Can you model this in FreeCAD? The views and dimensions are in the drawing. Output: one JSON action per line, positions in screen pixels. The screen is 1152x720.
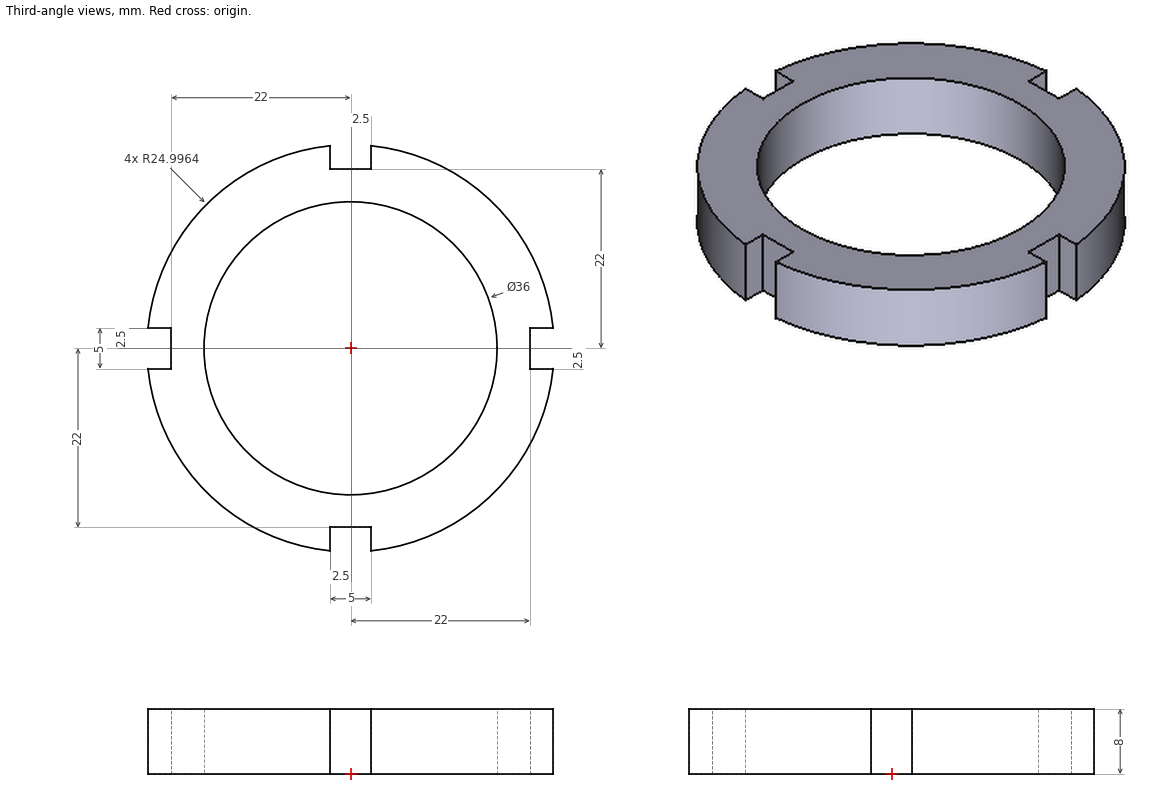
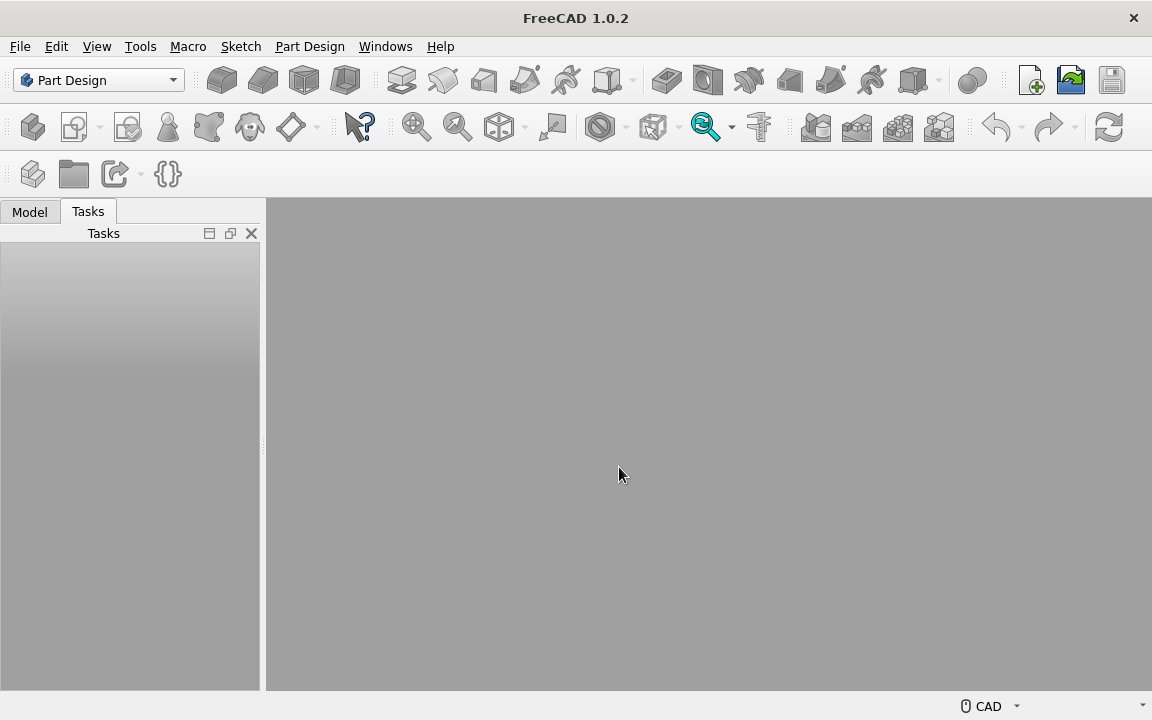
{"action": "key", "text": "ctrl+n"}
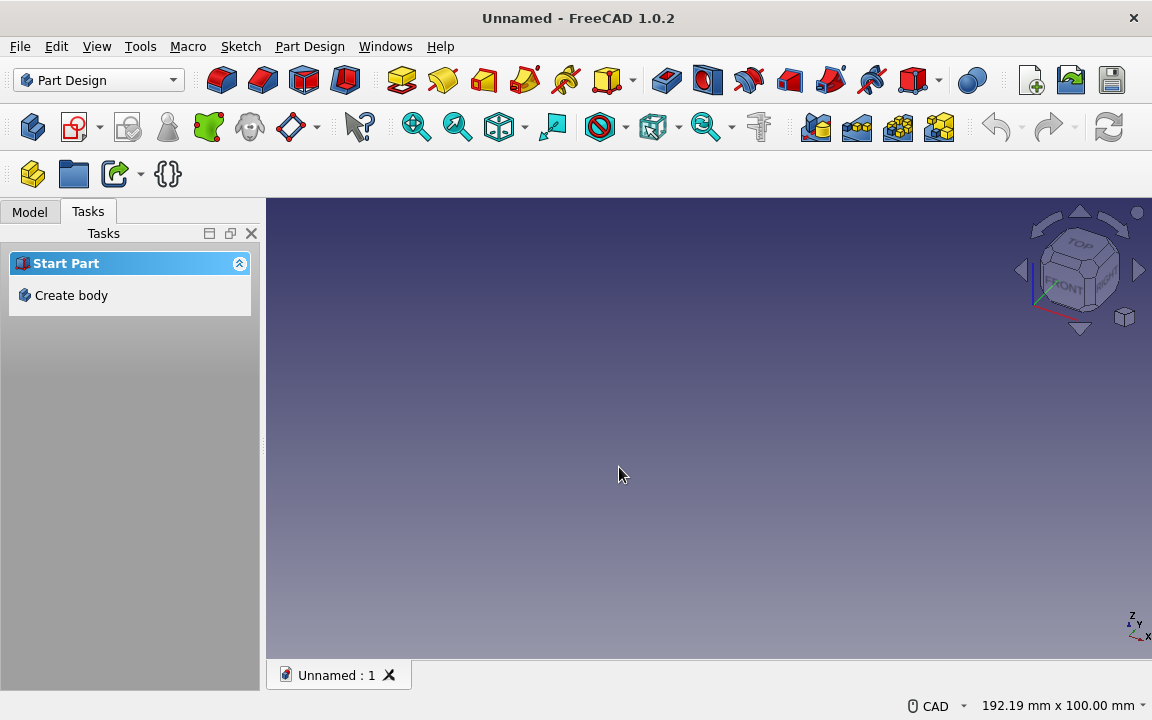
{"action": "left_click", "coordinate": [74, 128]}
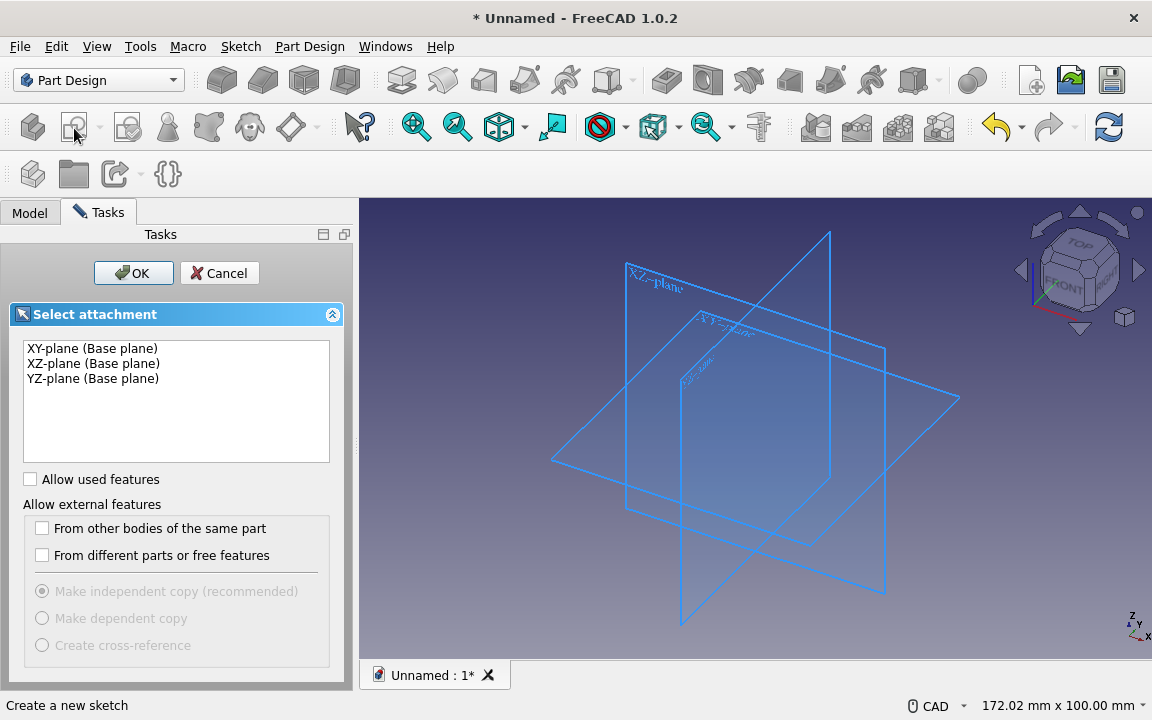
{"action": "left_click", "coordinate": [84, 348]}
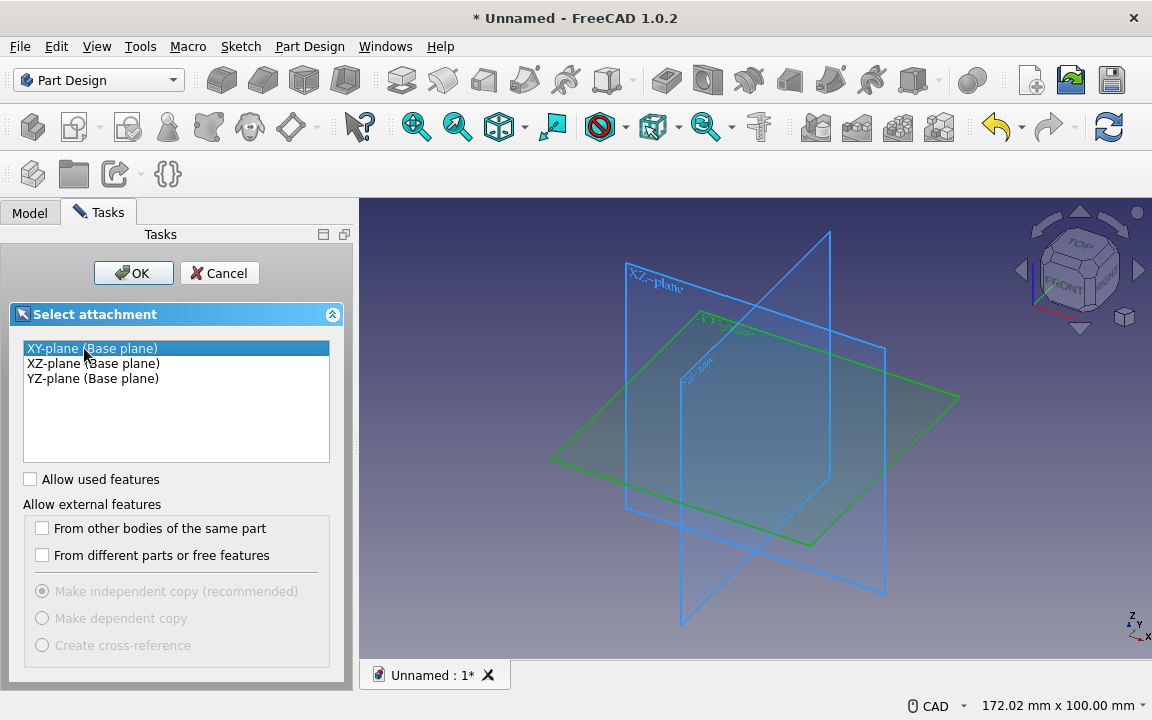
{"action": "left_click", "coordinate": [134, 273]}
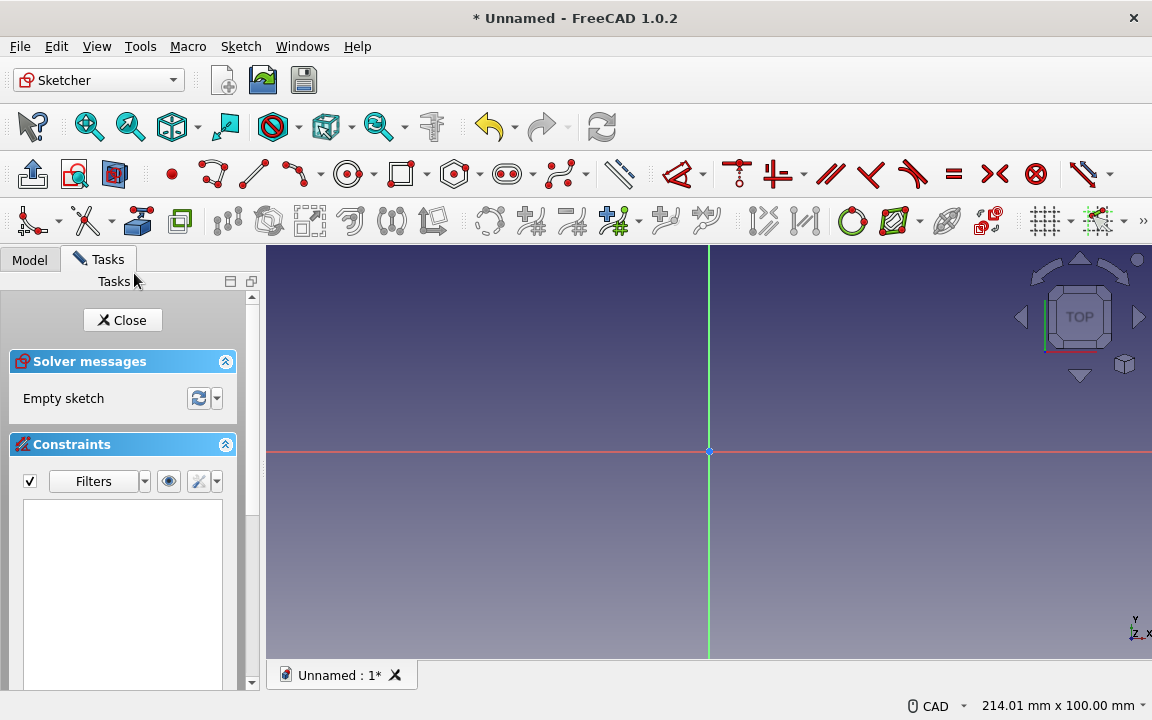
{"action": "key", "text": "g m"}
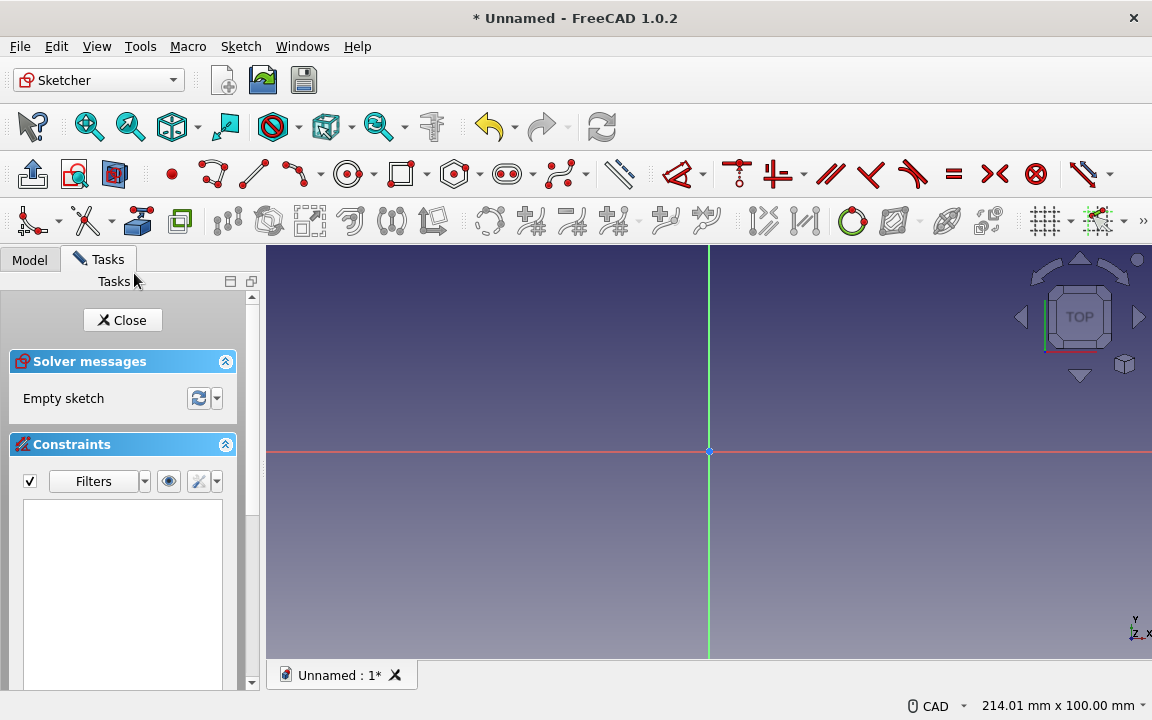
{"action": "scroll", "coordinate": [606, 442], "scroll_direction": "up", "scroll_amount": 3}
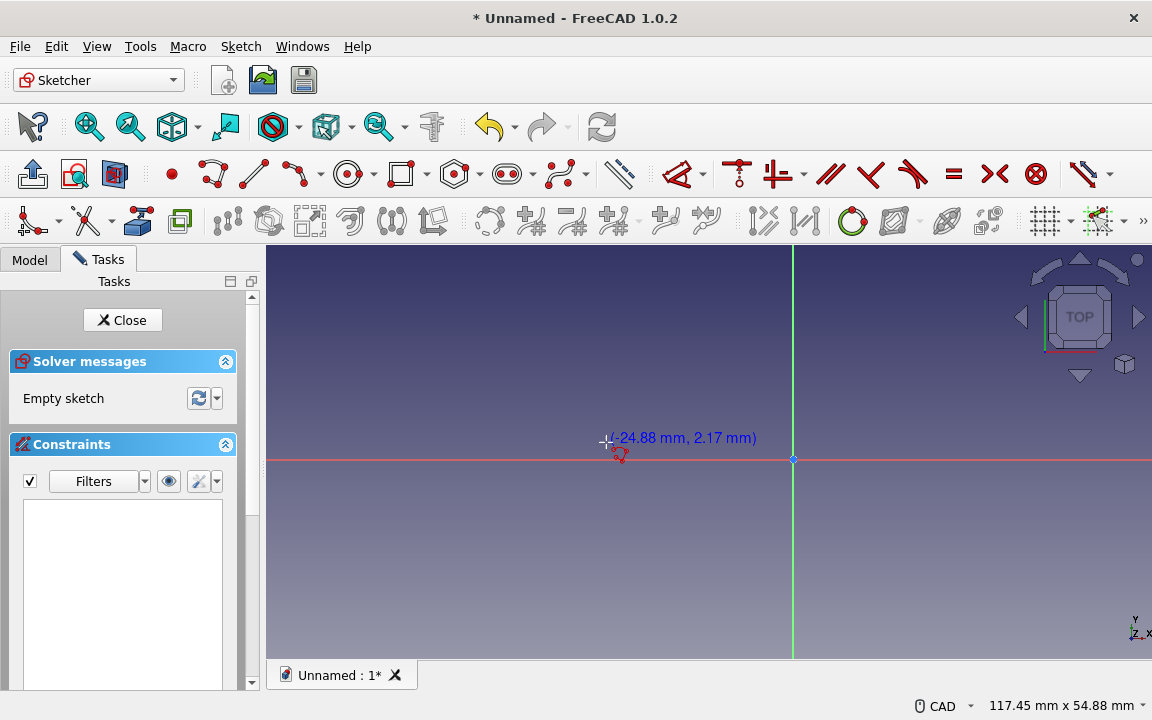
{"action": "left_click", "coordinate": [606, 441]}
{"action": "left_click", "coordinate": [627, 441]}
{"action": "left_click", "coordinate": [627, 479]}
{"action": "left_click", "coordinate": [606, 479]}
{"action": "right_click", "coordinate": [606, 479]}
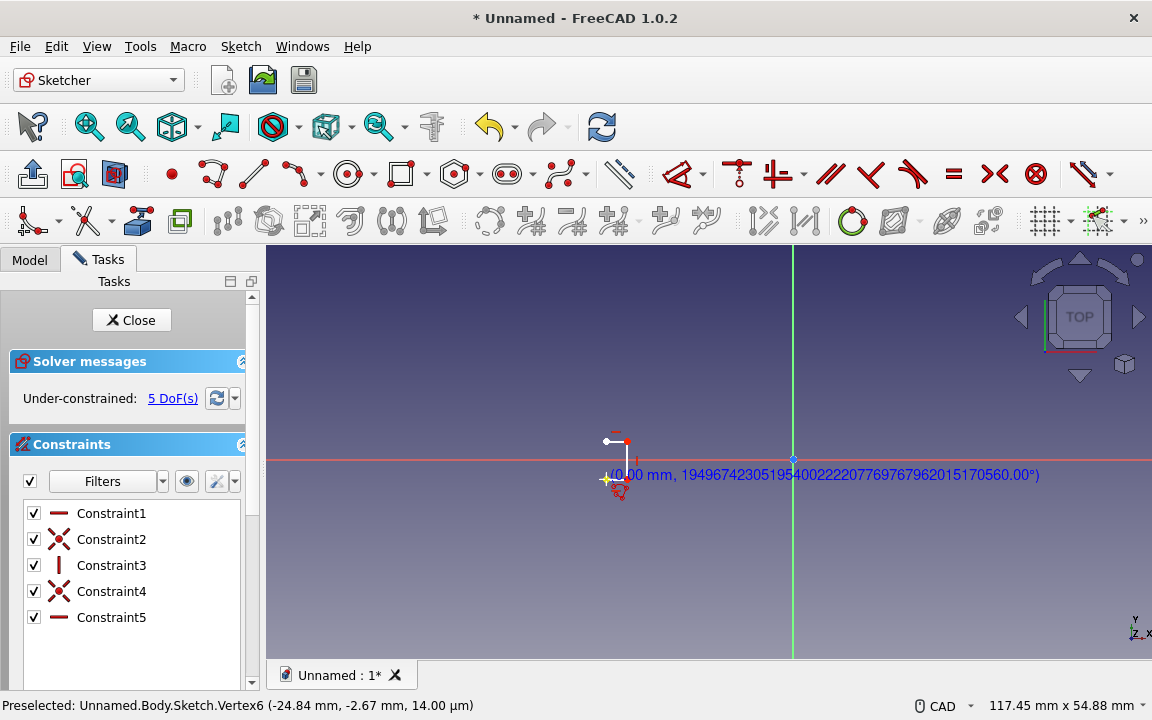
{"action": "scroll", "coordinate": [330, 436], "scroll_direction": "down", "scroll_amount": 2}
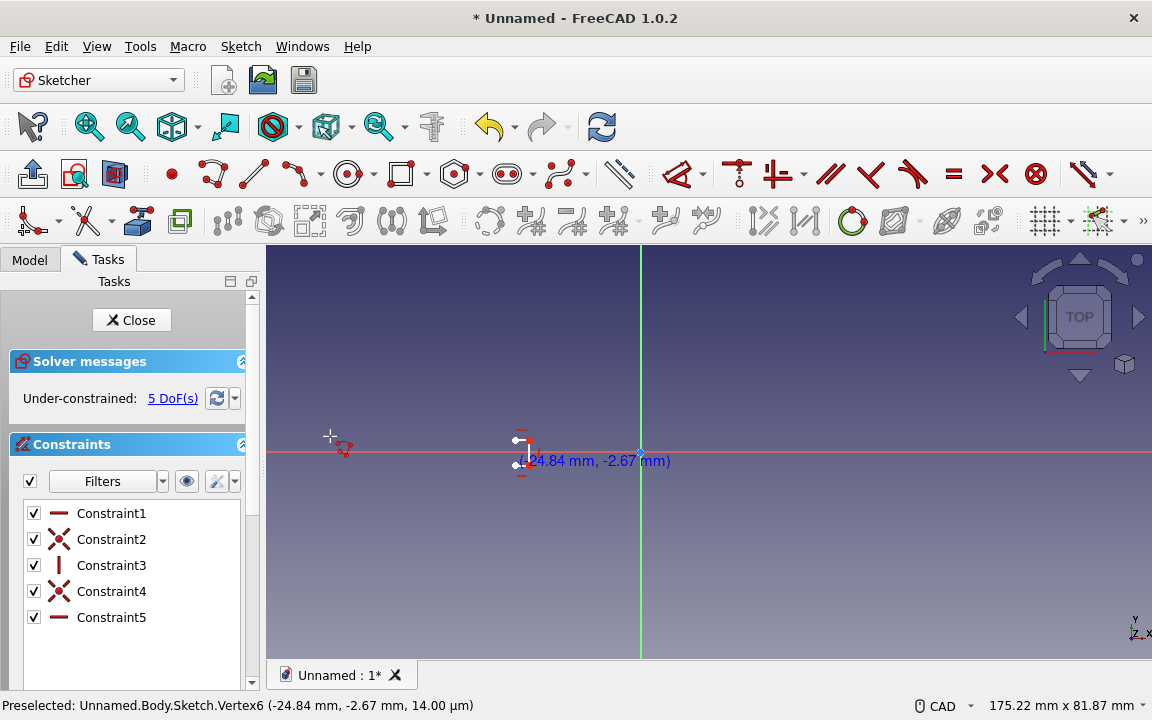
{"action": "scroll", "coordinate": [628, 578], "scroll_direction": "up", "scroll_amount": 2}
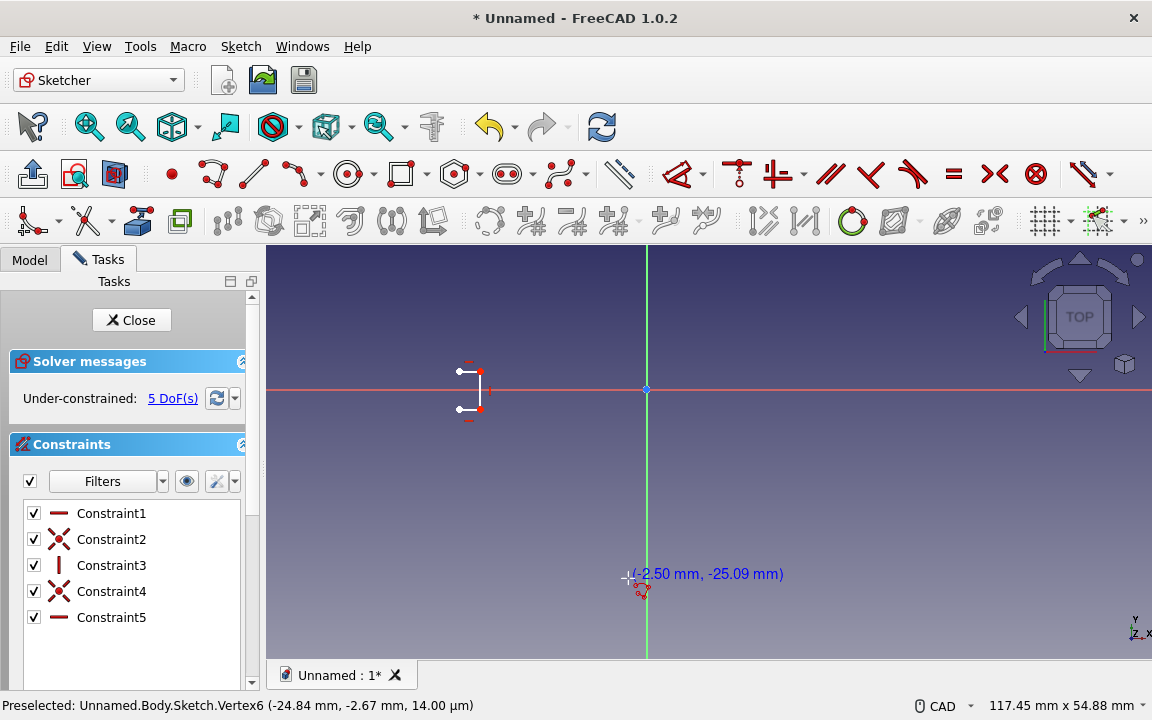
{"action": "left_click", "coordinate": [628, 577]}
{"action": "left_click", "coordinate": [628, 556]}
{"action": "left_click", "coordinate": [665, 556]}
{"action": "left_click", "coordinate": [665, 577]}
{"action": "right_click", "coordinate": [665, 577]}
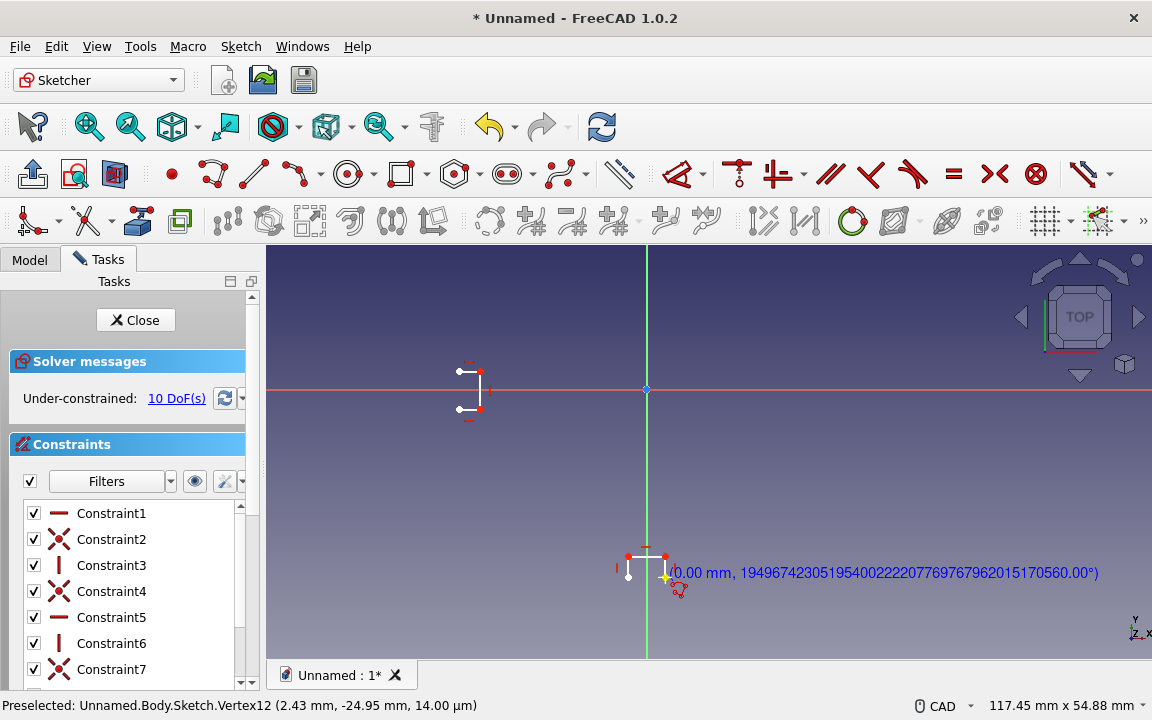
{"action": "left_click", "coordinate": [834, 409]}
{"action": "left_click", "coordinate": [813, 409]}
{"action": "left_click", "coordinate": [813, 371]}
{"action": "left_click", "coordinate": [834, 371]}
{"action": "right_click", "coordinate": [834, 371]}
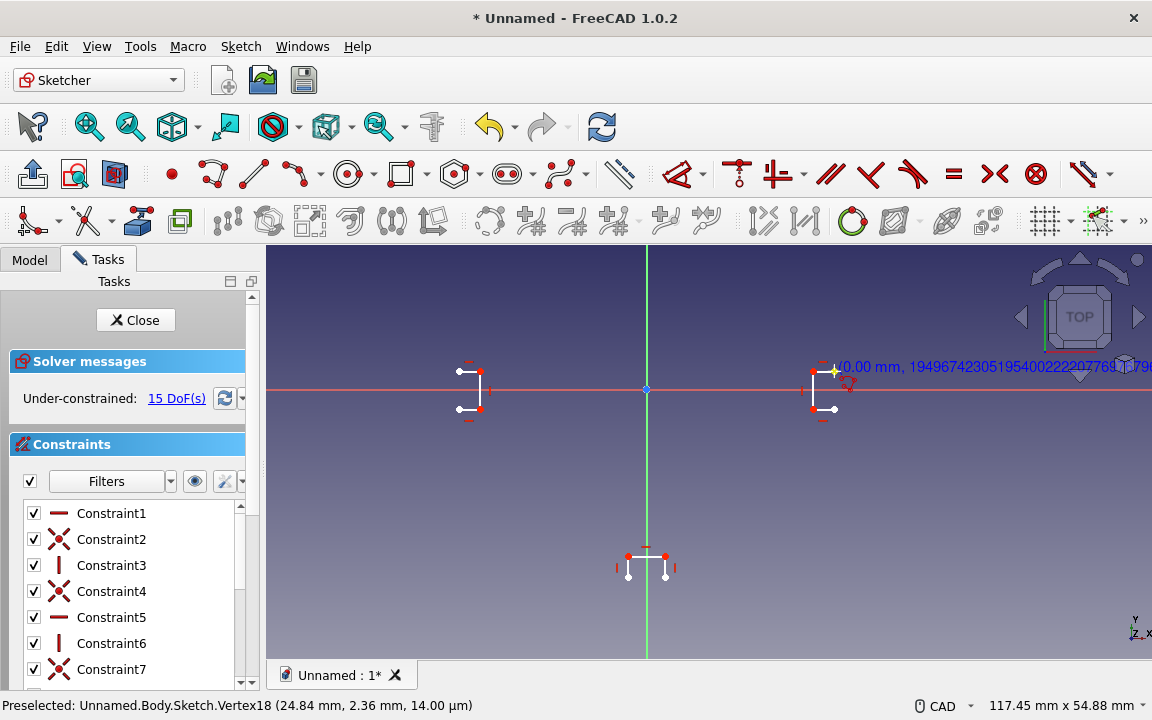
{"action": "scroll", "coordinate": [628, 578], "scroll_direction": "down", "scroll_amount": 2}